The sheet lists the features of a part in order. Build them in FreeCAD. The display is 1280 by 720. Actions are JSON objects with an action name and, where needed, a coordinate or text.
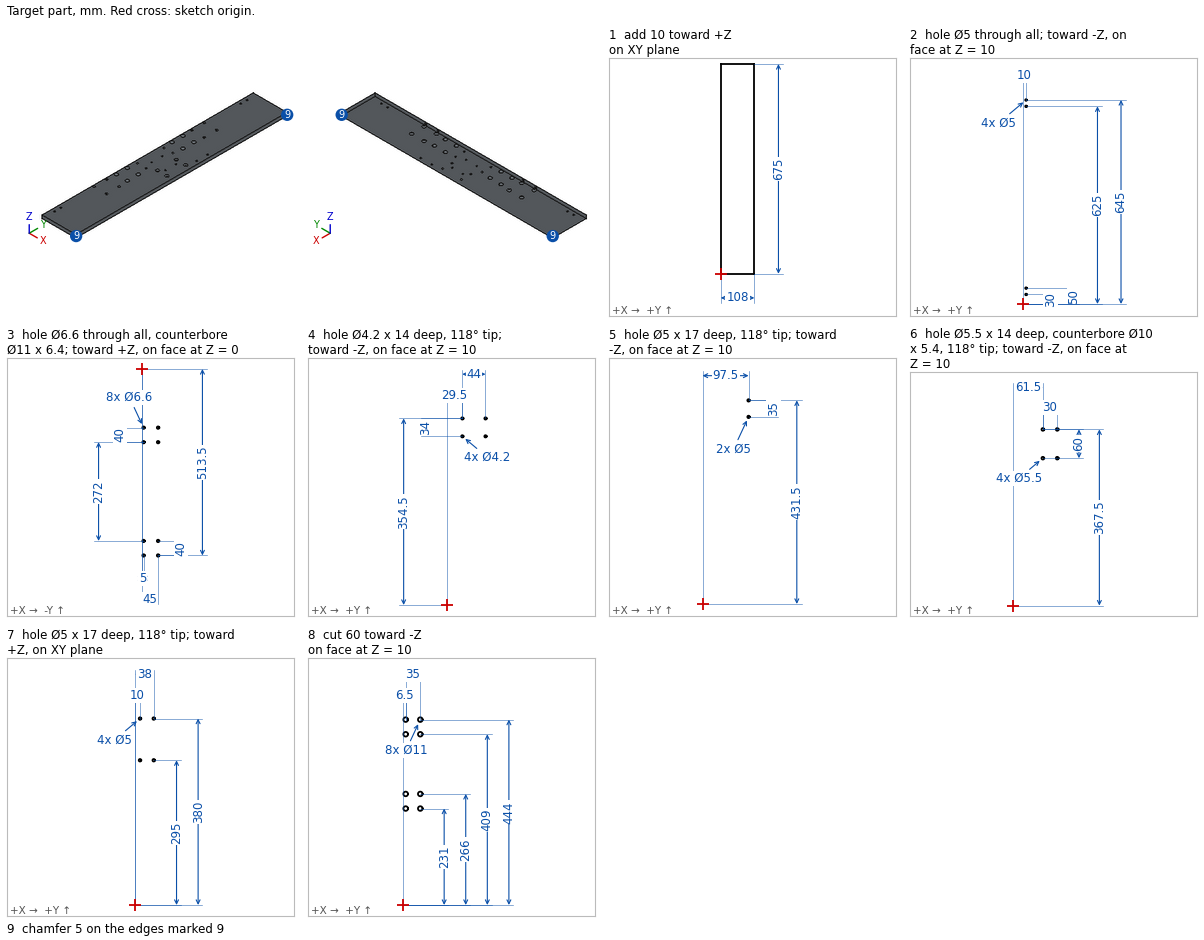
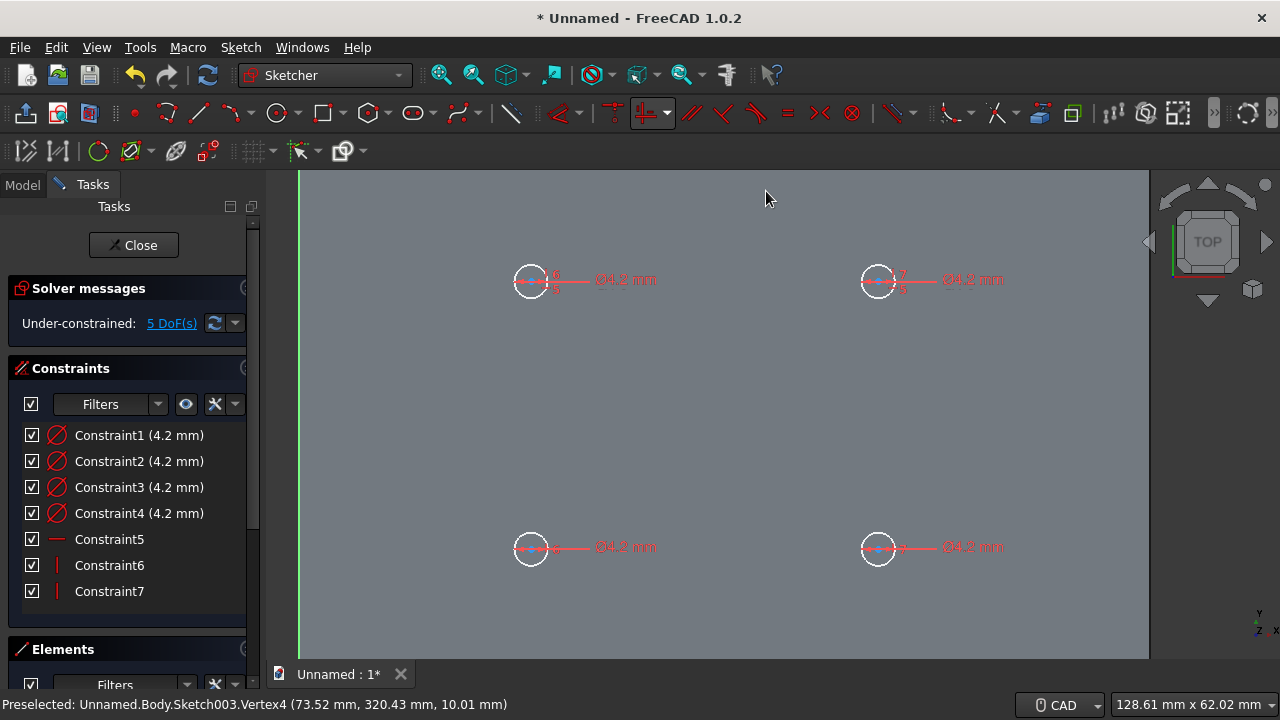
{"action": "left_click", "coordinate": [531, 549]}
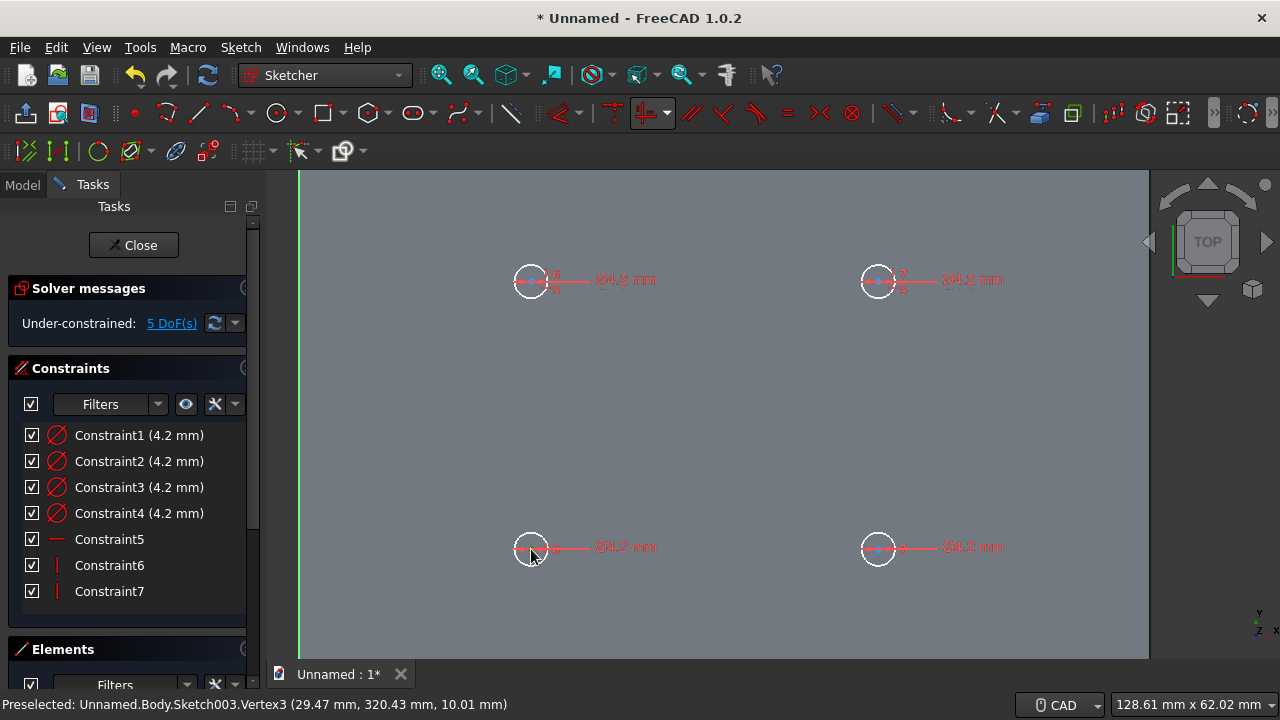
{"action": "left_click", "coordinate": [878, 549]}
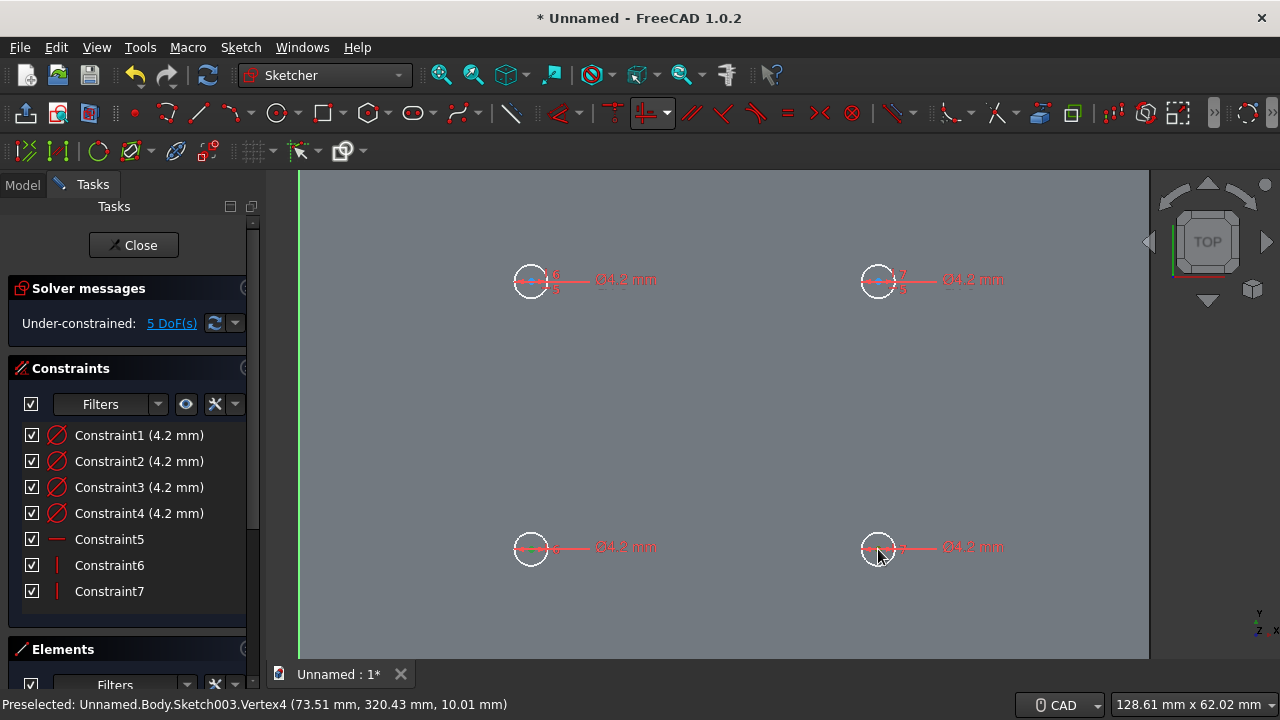
{"action": "left_click", "coordinate": [670, 114]}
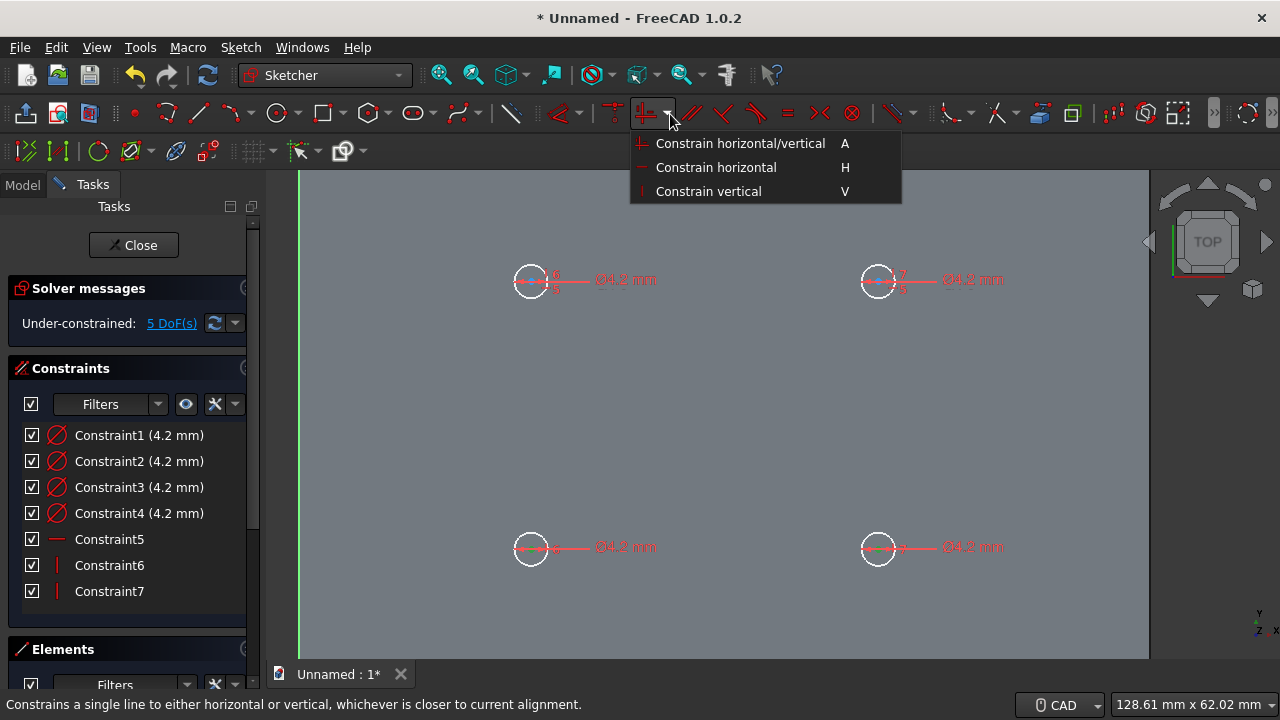
{"action": "left_click", "coordinate": [766, 167]}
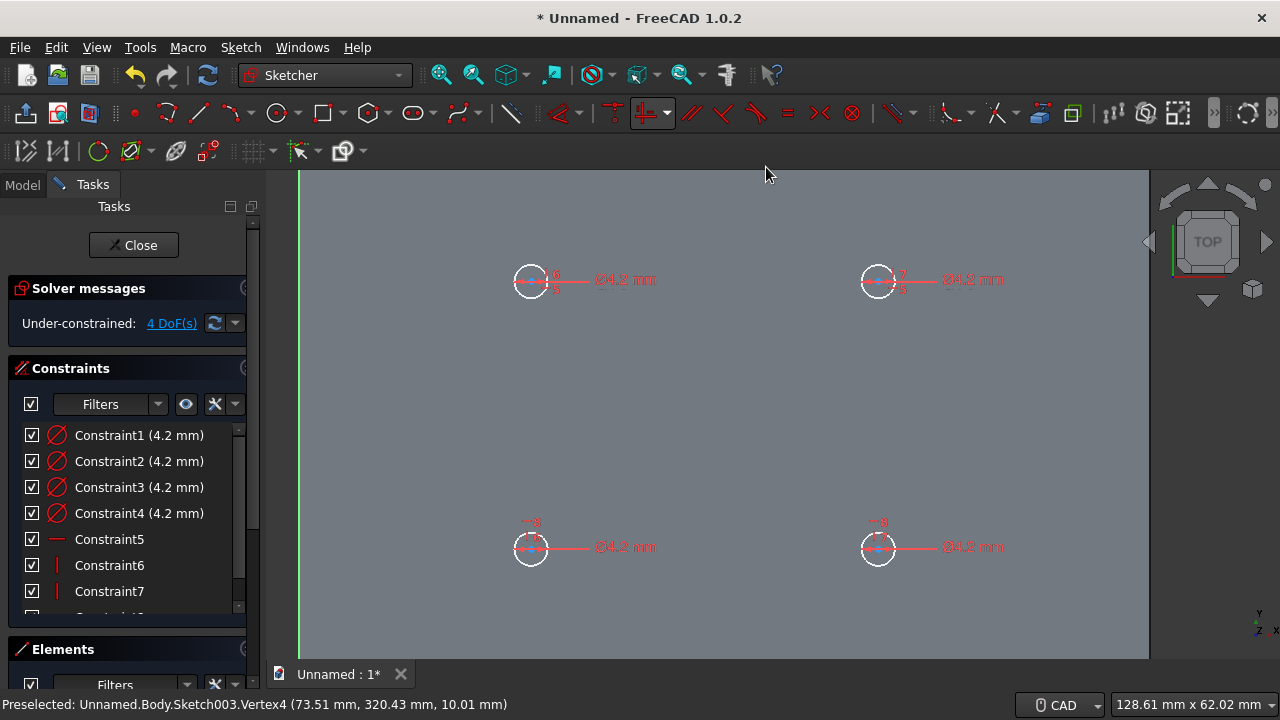
{"action": "key", "text": "d"}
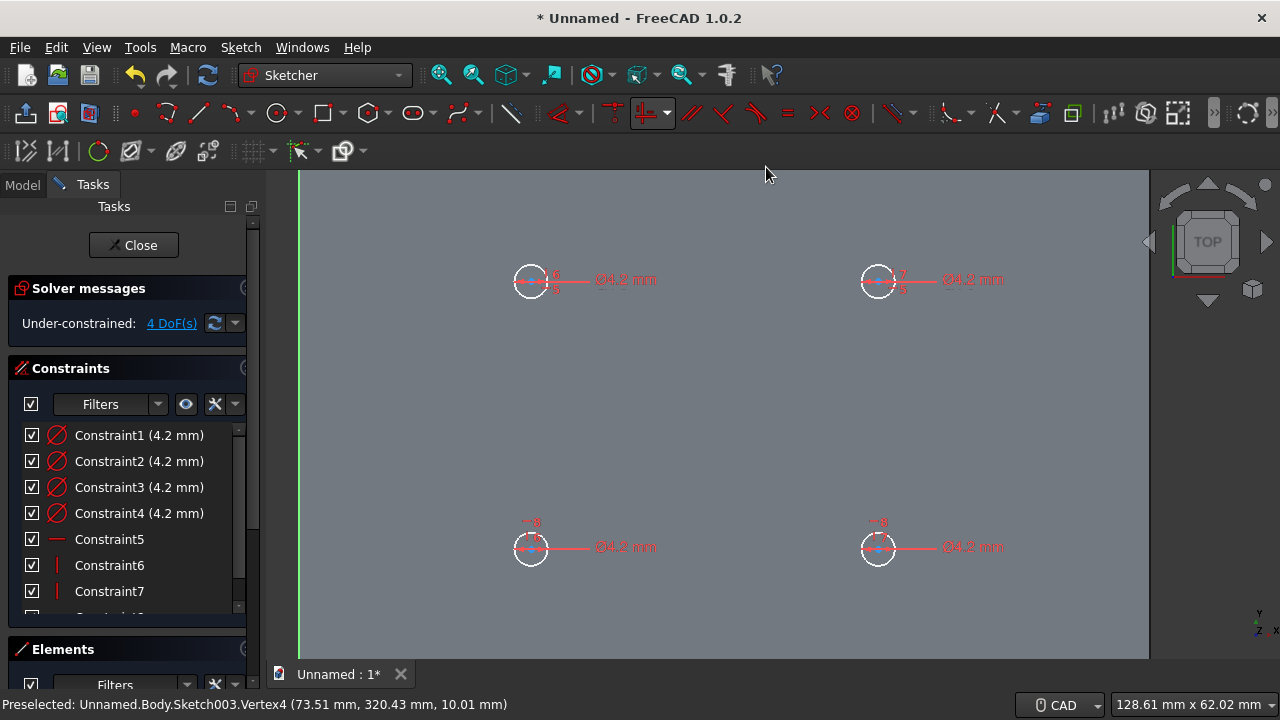
{"action": "left_click", "coordinate": [531, 282]}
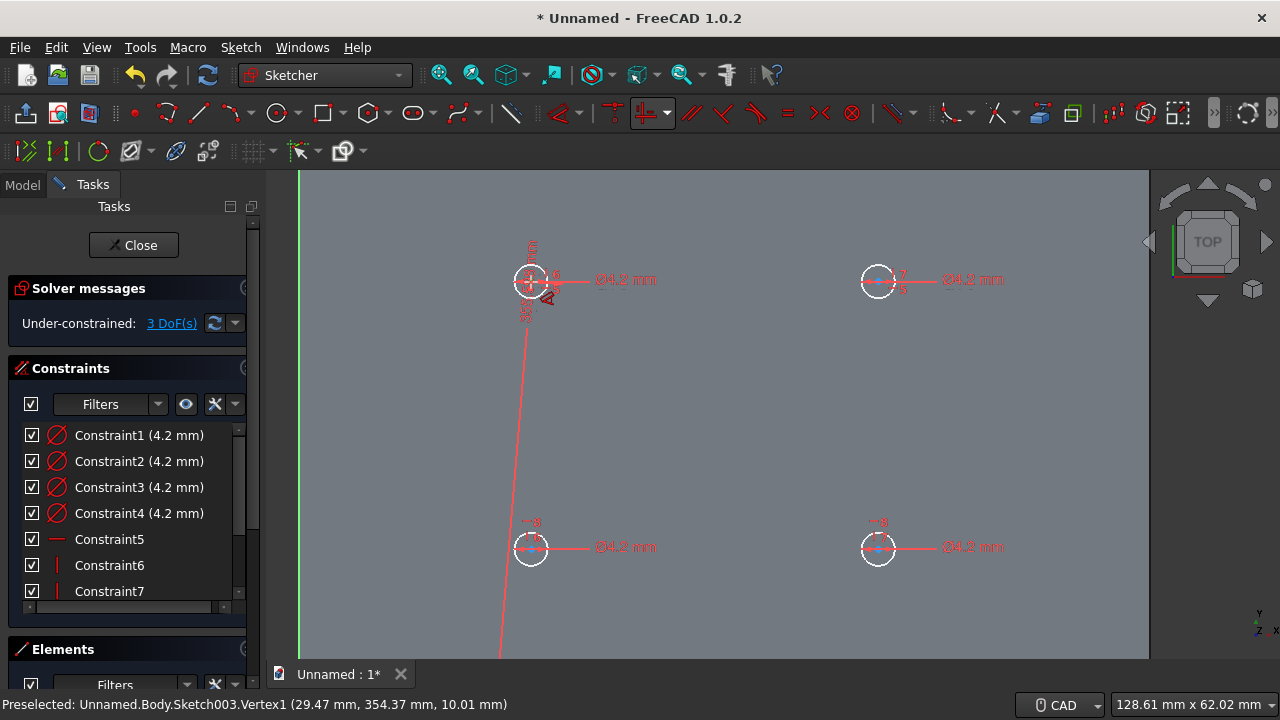
{"action": "left_click", "coordinate": [878, 282]}
{"action": "left_click", "coordinate": [705, 248]}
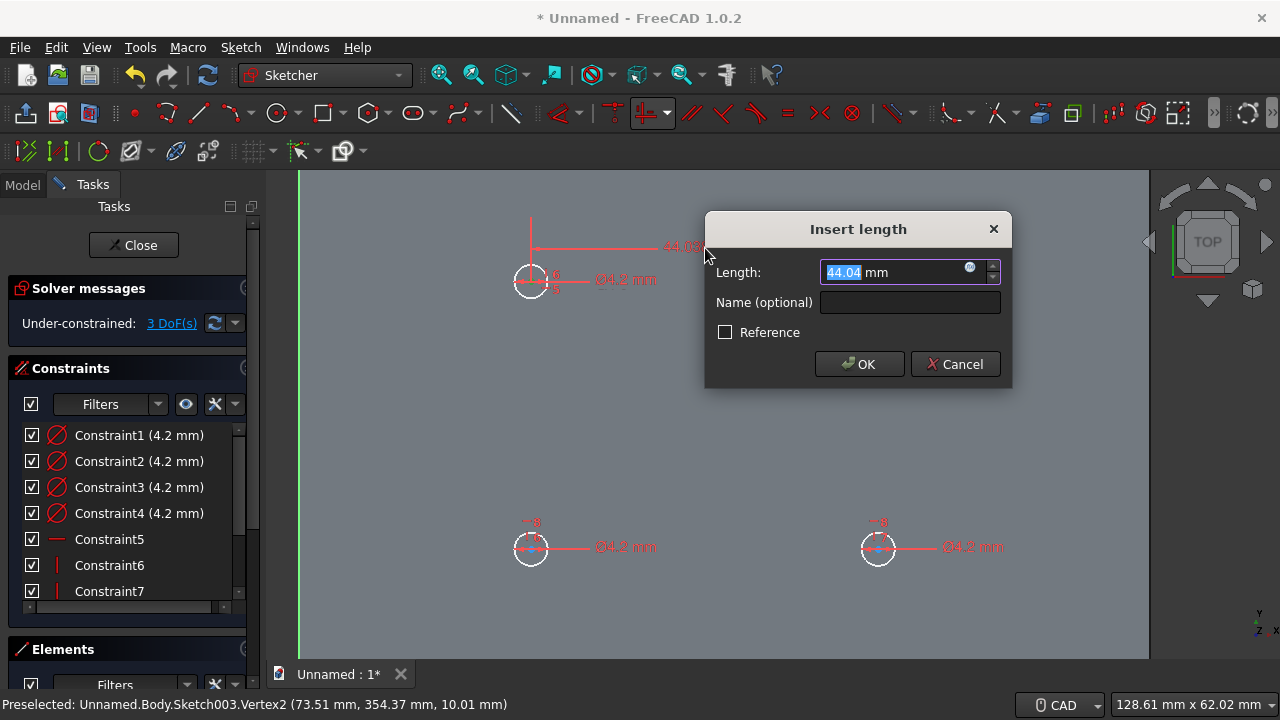
{"action": "type", "text": "44"}
{"action": "key", "text": "Return"}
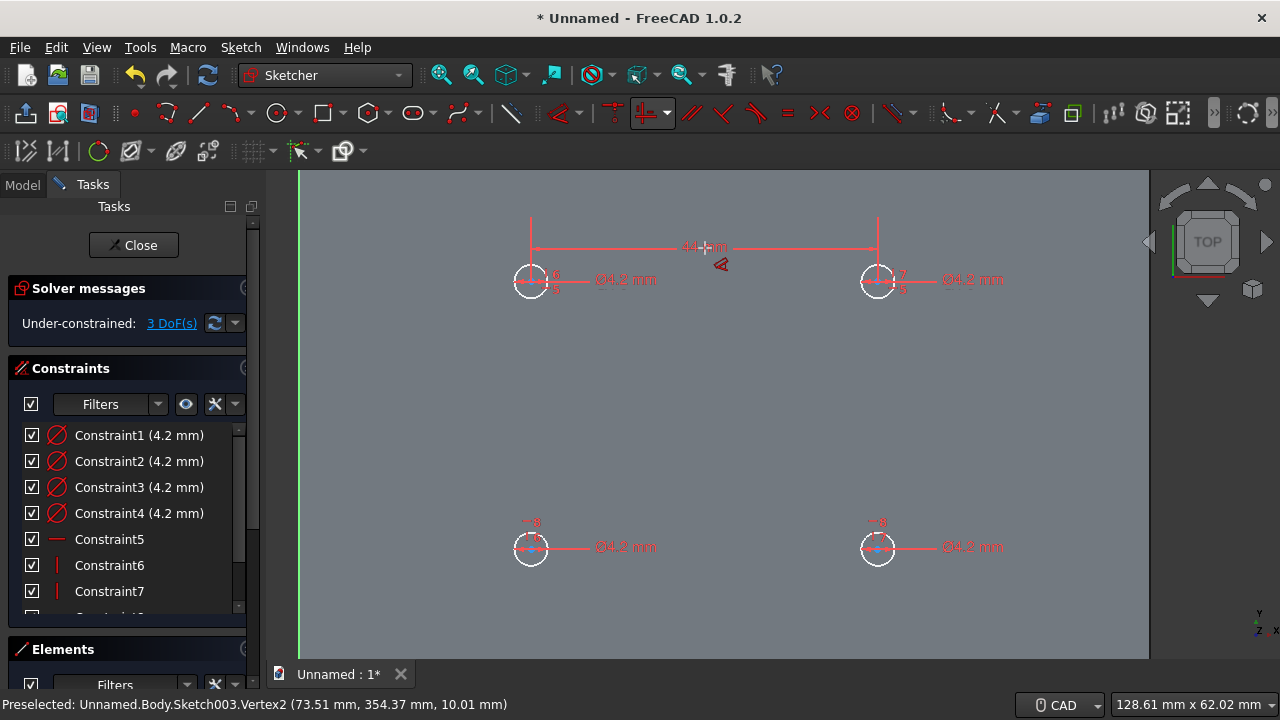
{"action": "left_click", "coordinate": [531, 282]}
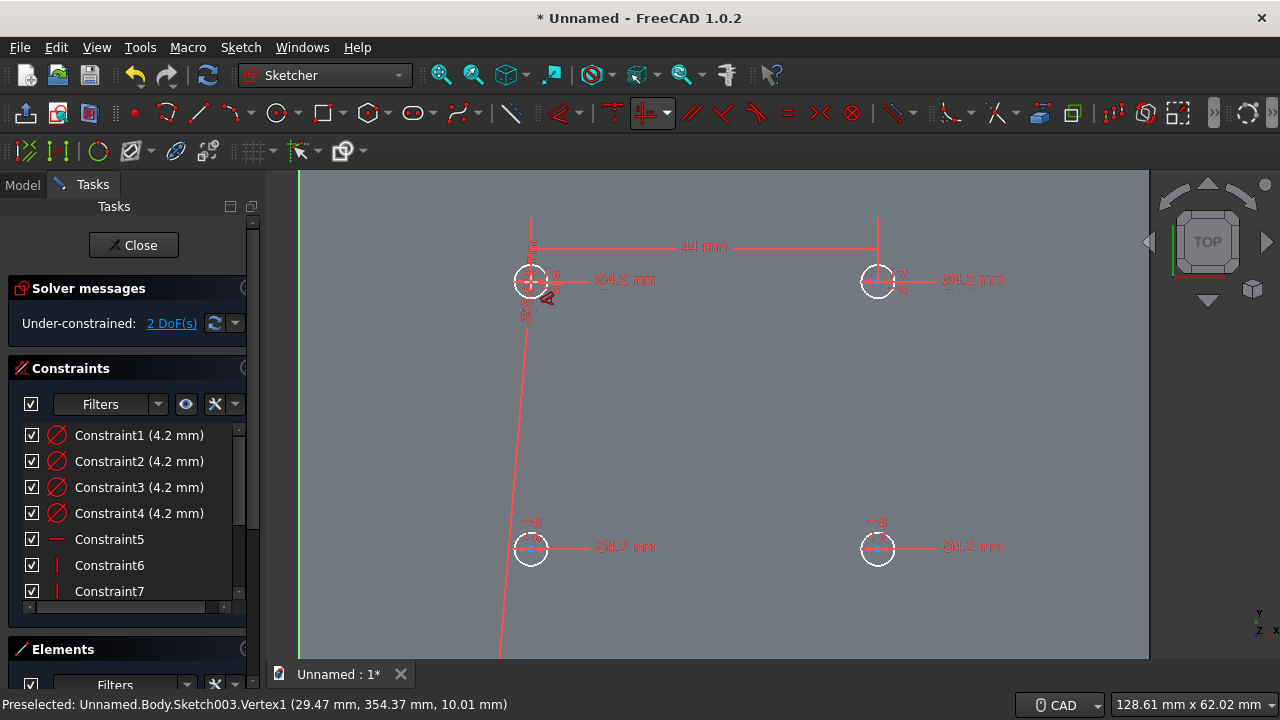
{"action": "left_click", "coordinate": [531, 549]}
{"action": "left_click", "coordinate": [497, 415]}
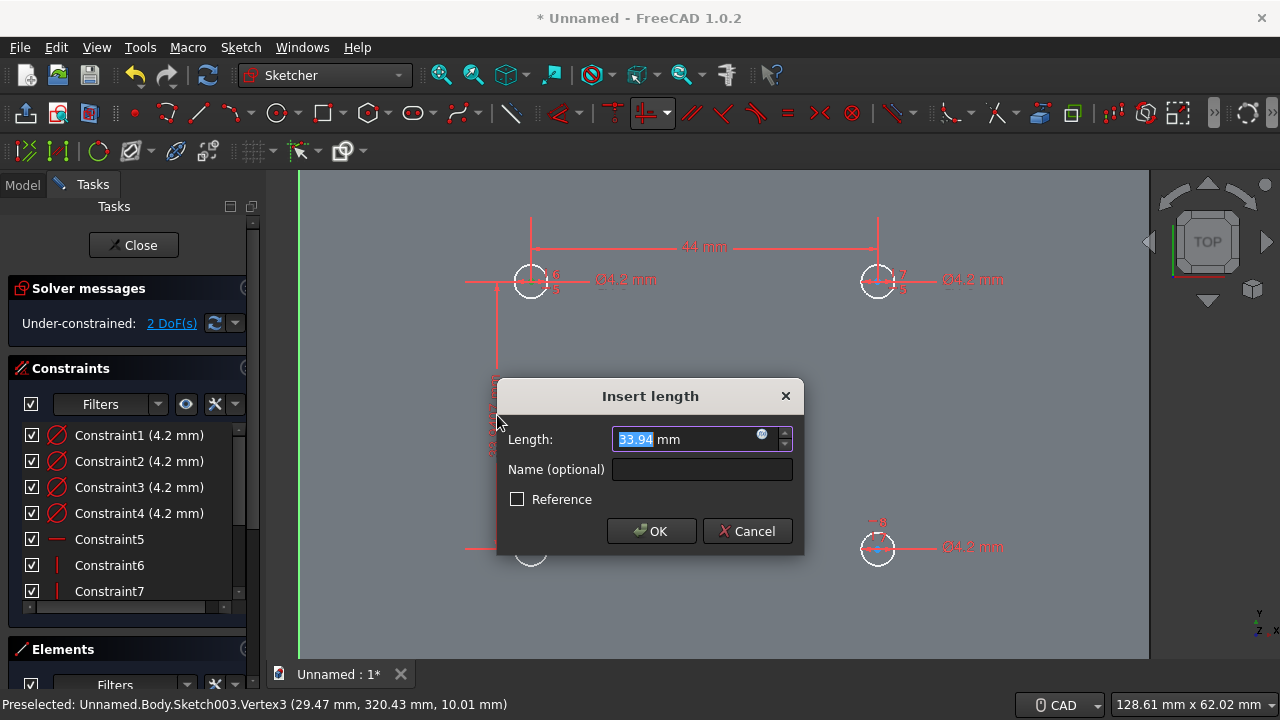
{"action": "type", "text": "34"}
{"action": "key", "text": "Return"}